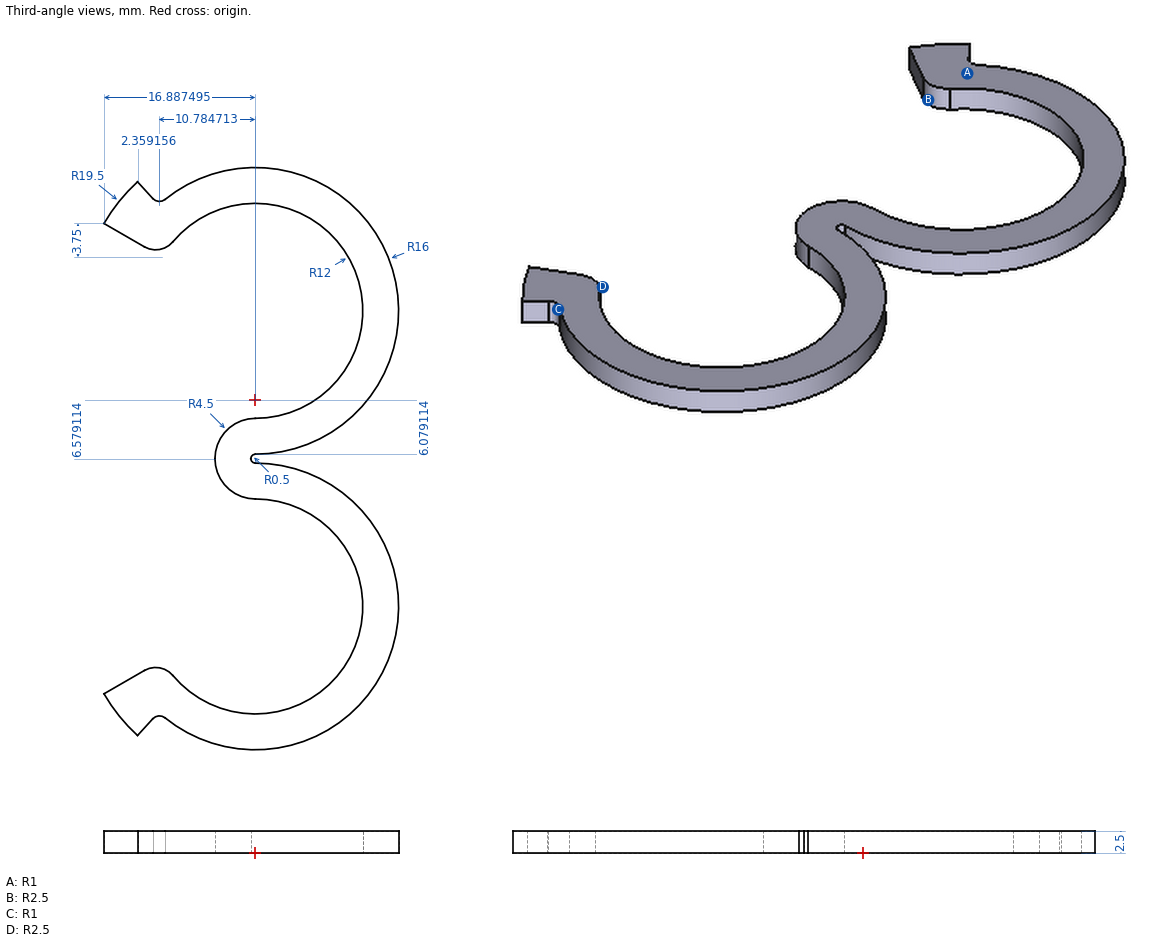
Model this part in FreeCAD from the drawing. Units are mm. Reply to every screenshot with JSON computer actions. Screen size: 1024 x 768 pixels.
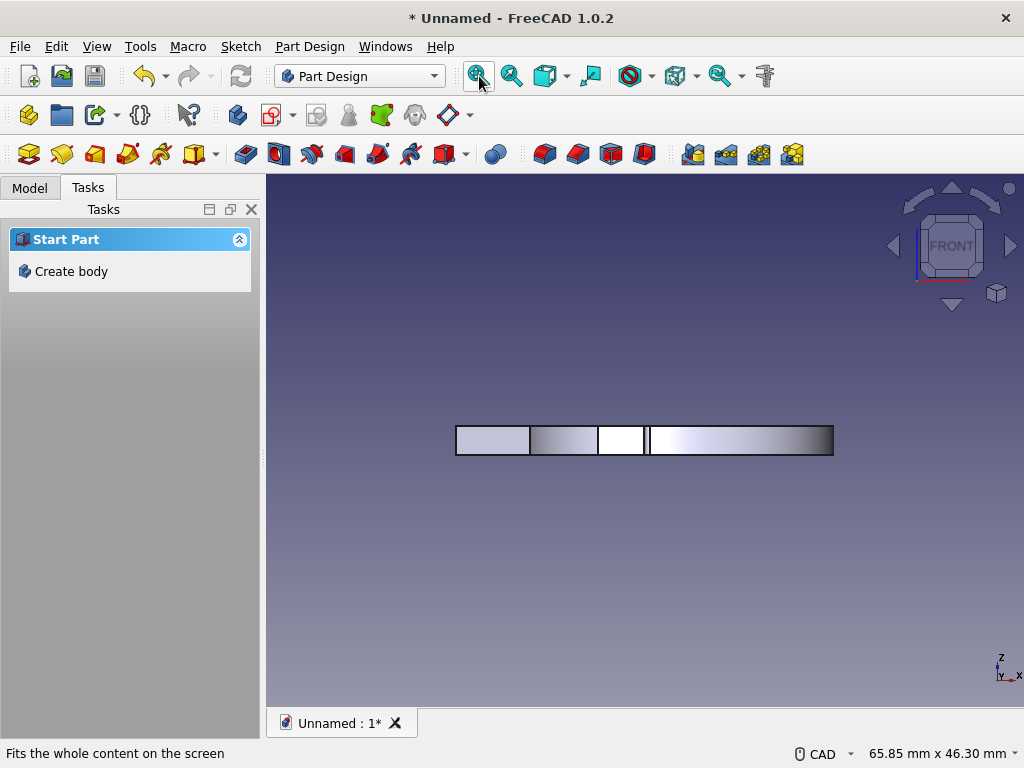
{"action": "key", "text": "3"}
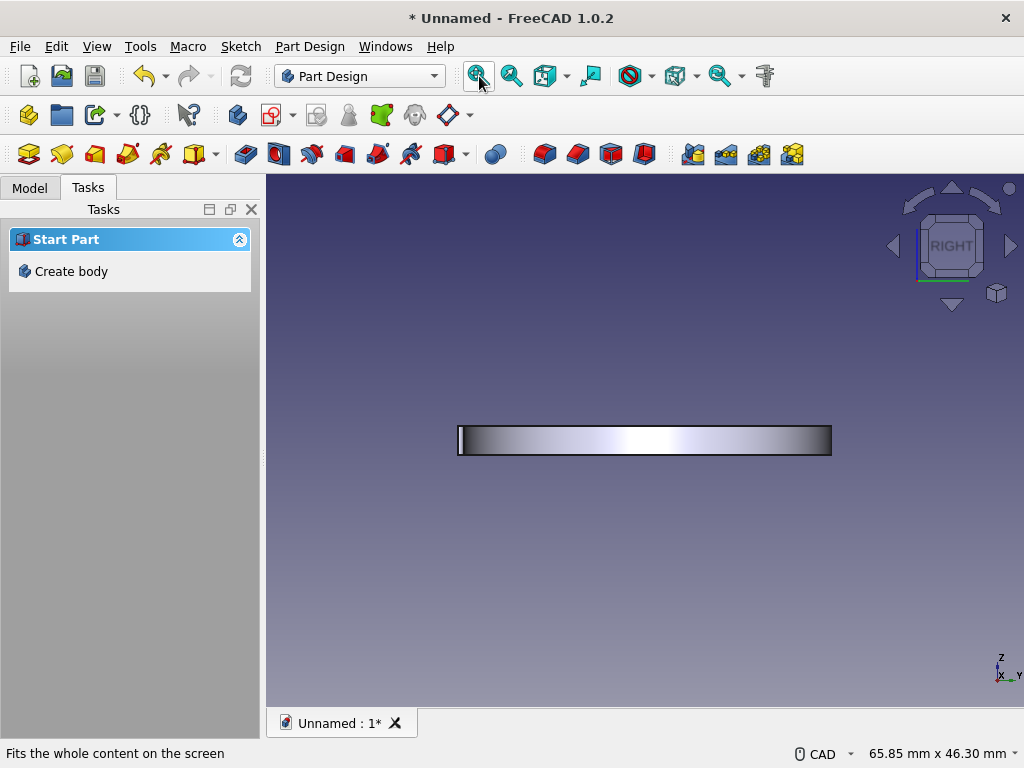
{"action": "key", "text": "5"}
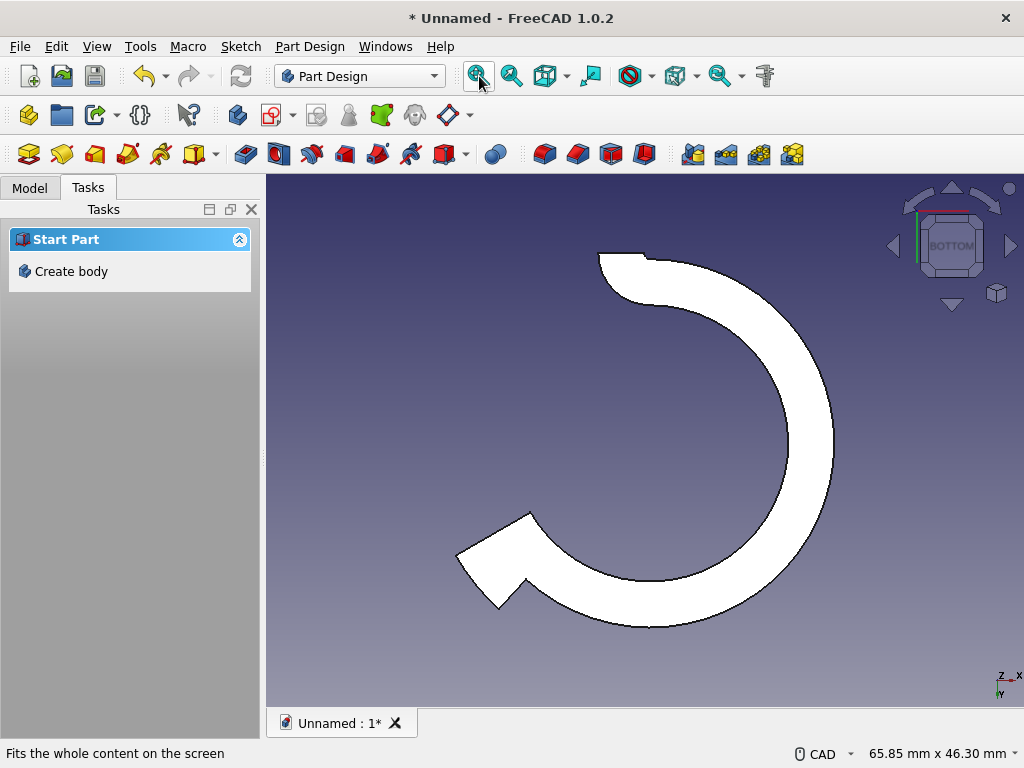
{"action": "key", "text": "4"}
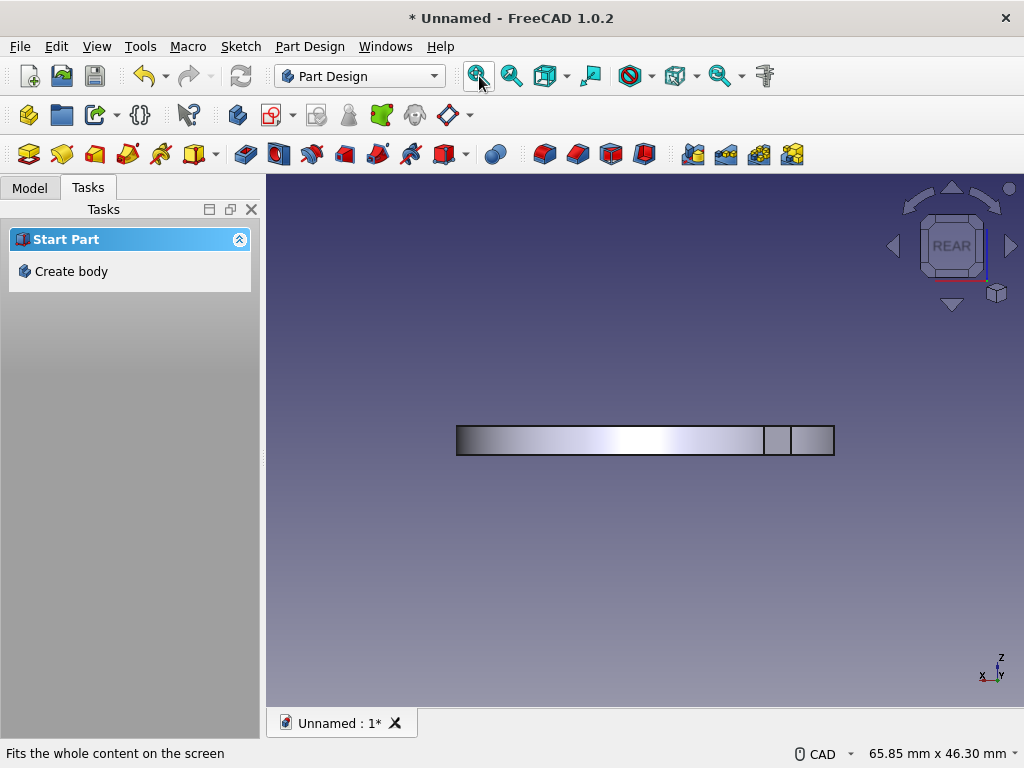
{"action": "key", "text": "6"}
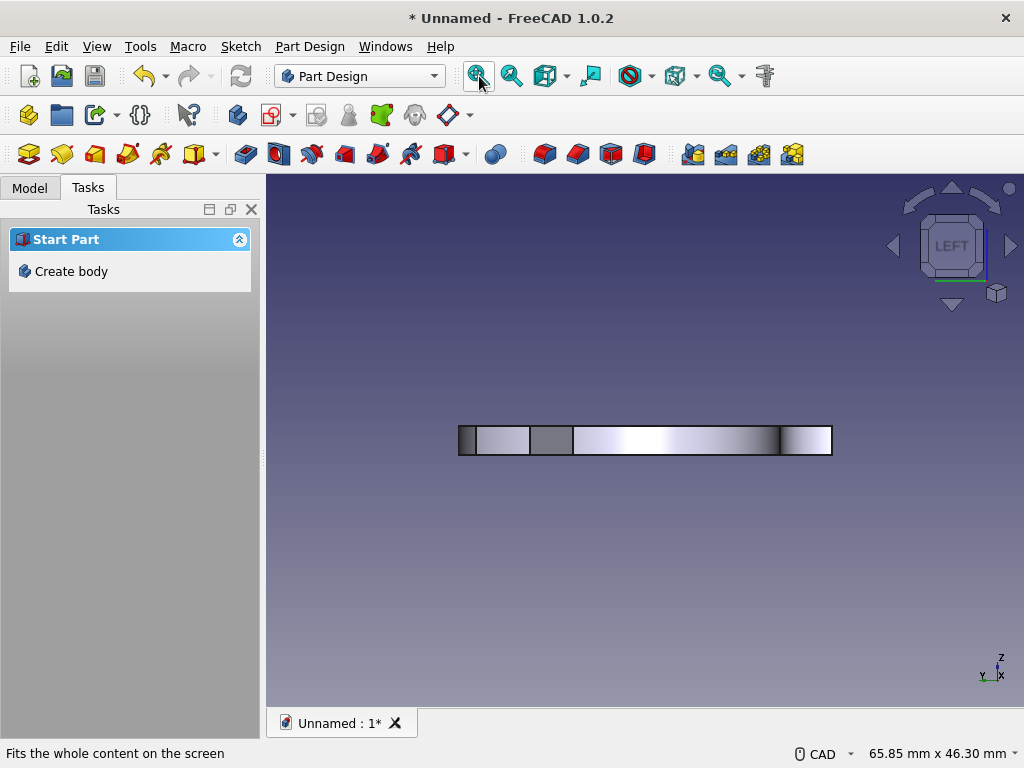
{"action": "key", "text": "v 3"}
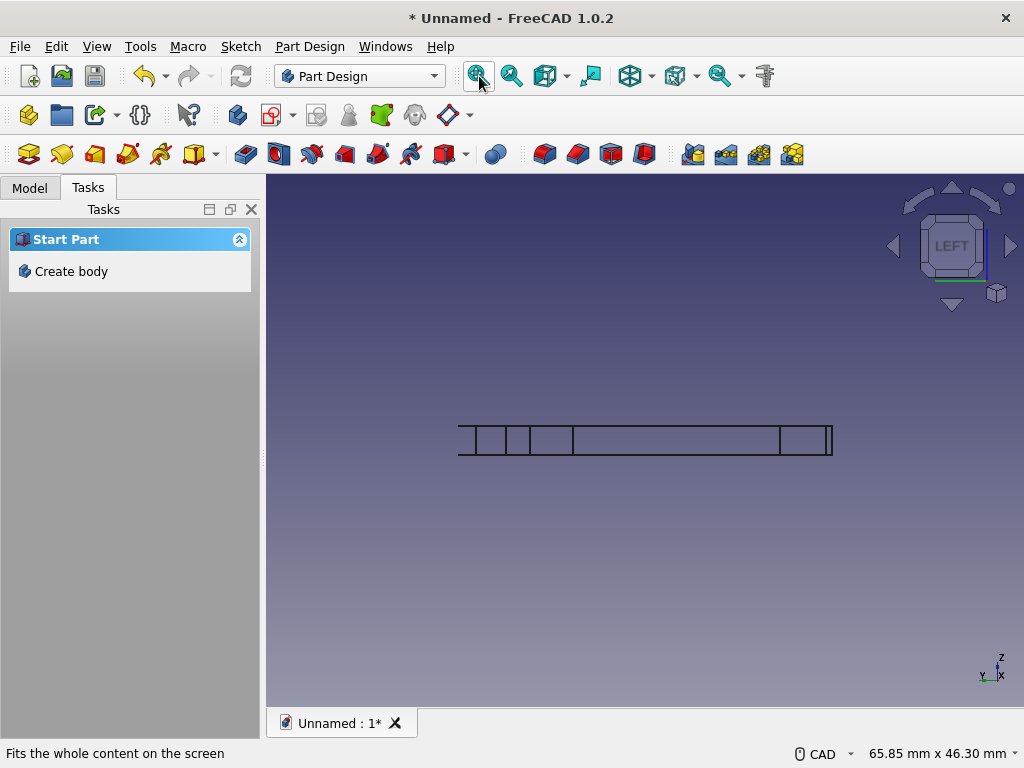
{"action": "key", "text": "0"}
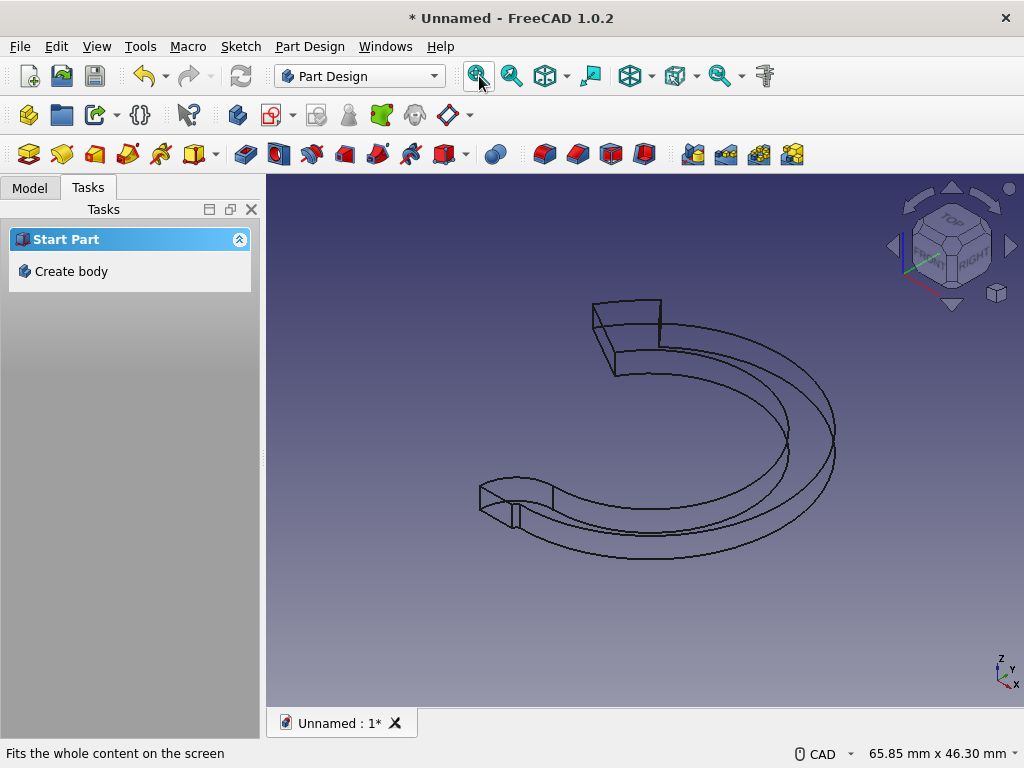
{"action": "left_click", "coordinate": [659, 334]}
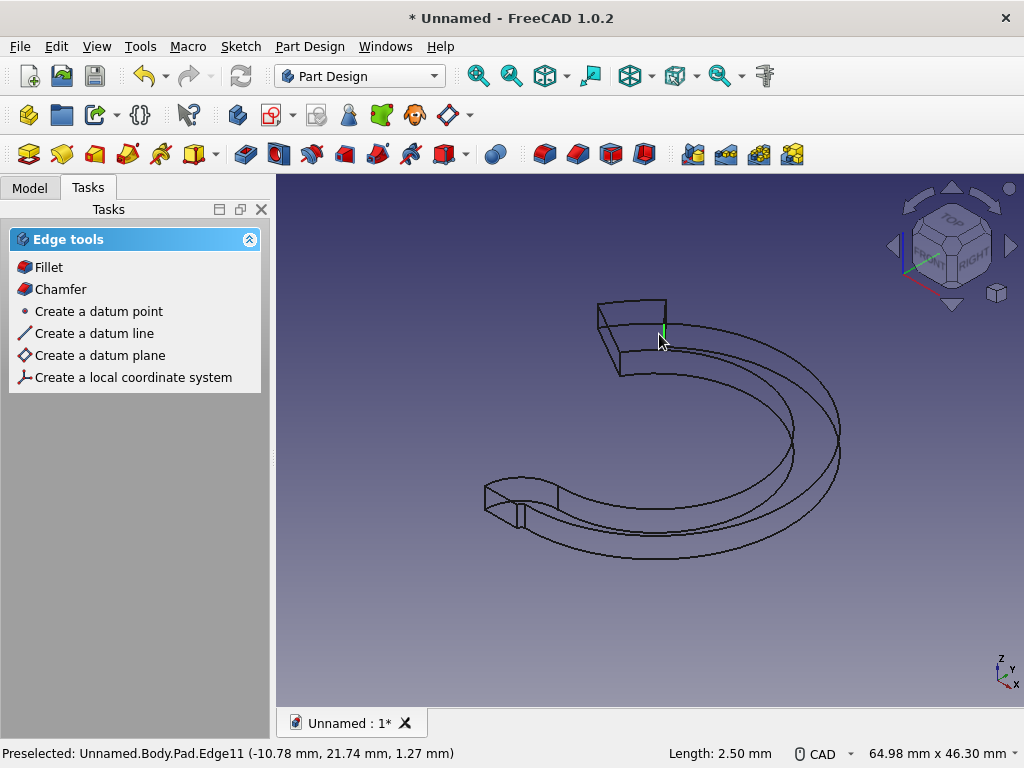
{"action": "key", "text": "v 1"}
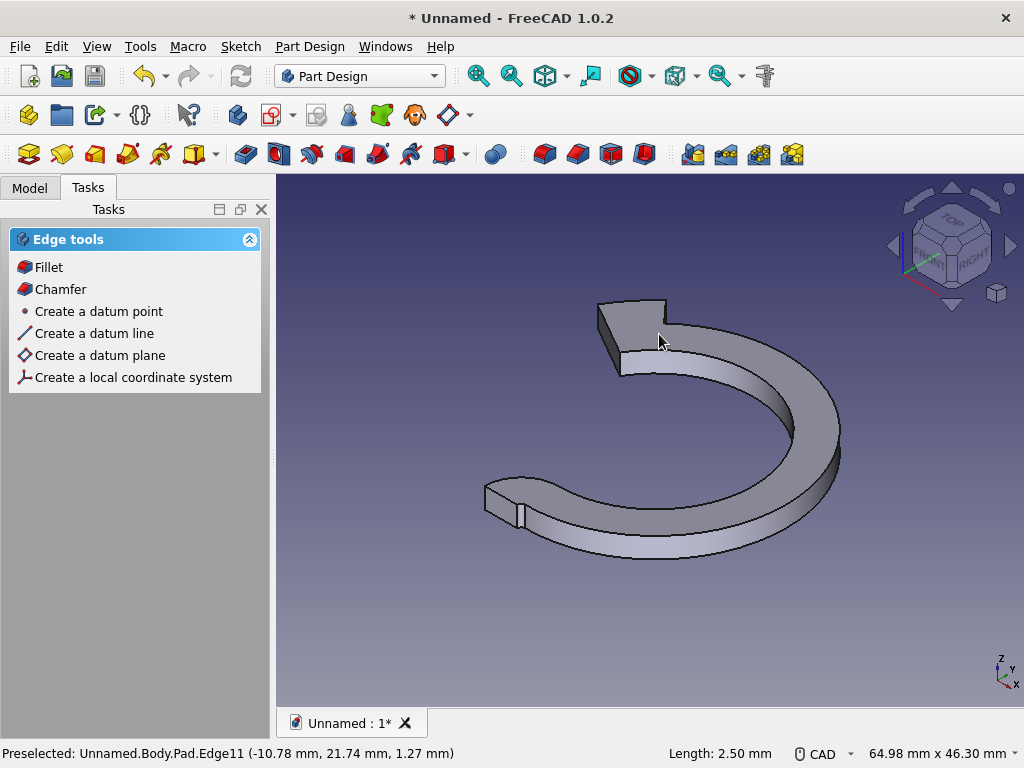
{"action": "left_click", "coordinate": [545, 154]}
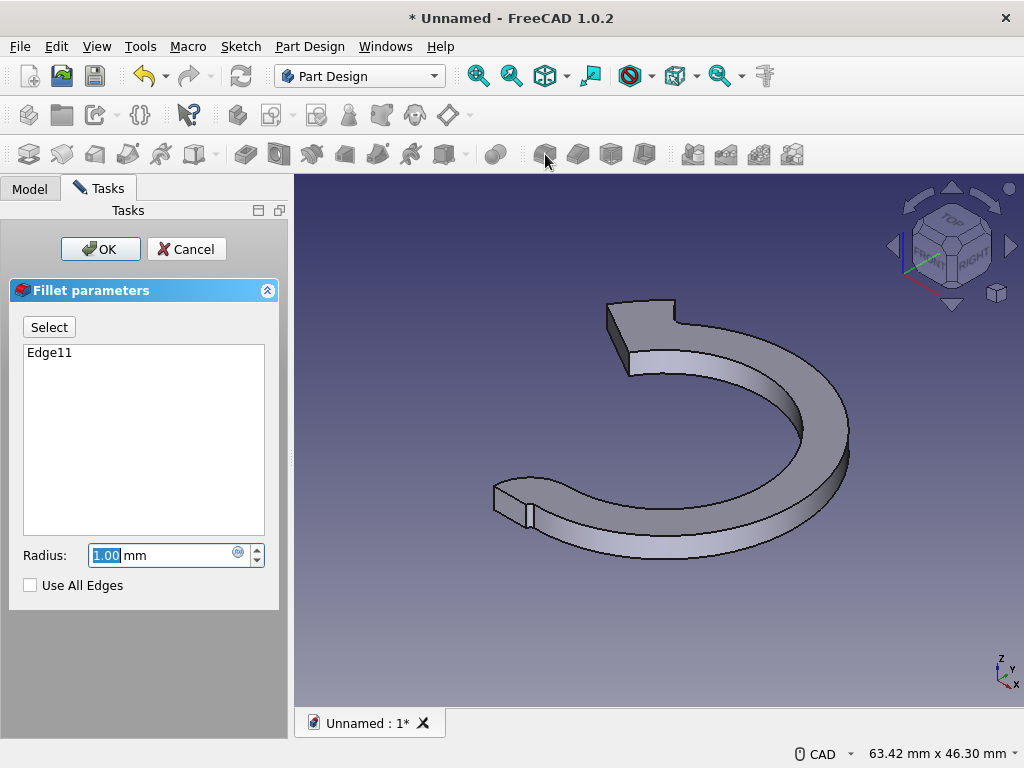
{"action": "type", "text": "1"}
{"action": "key", "text": "Tab"}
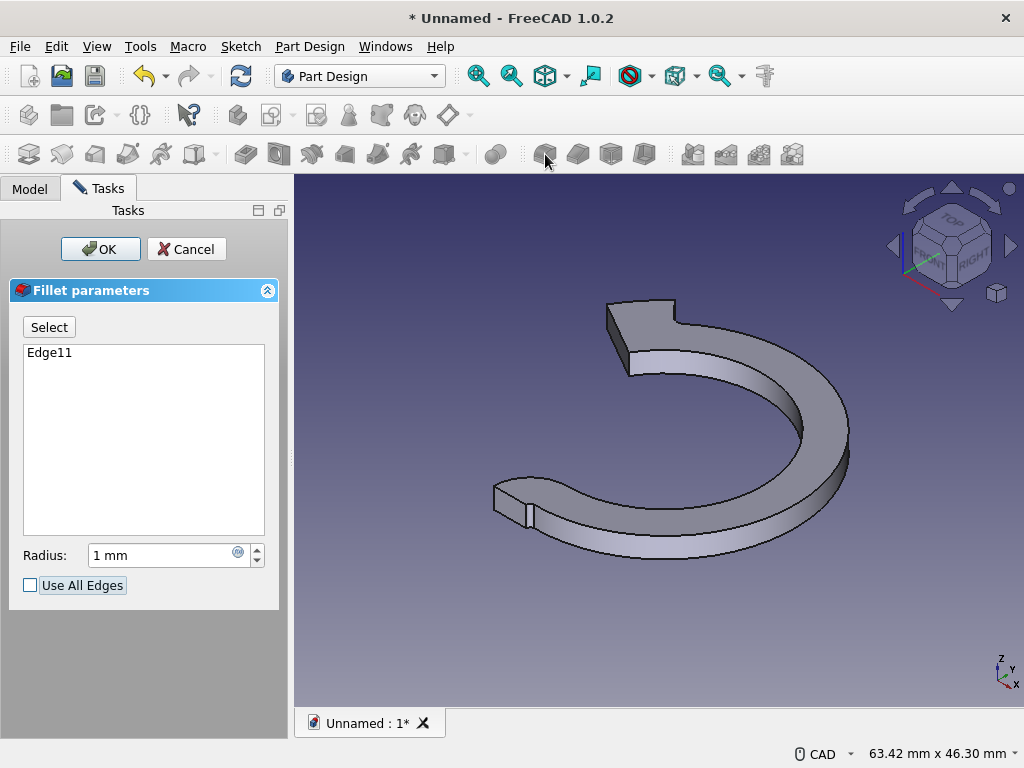
{"action": "left_click", "coordinate": [101, 249]}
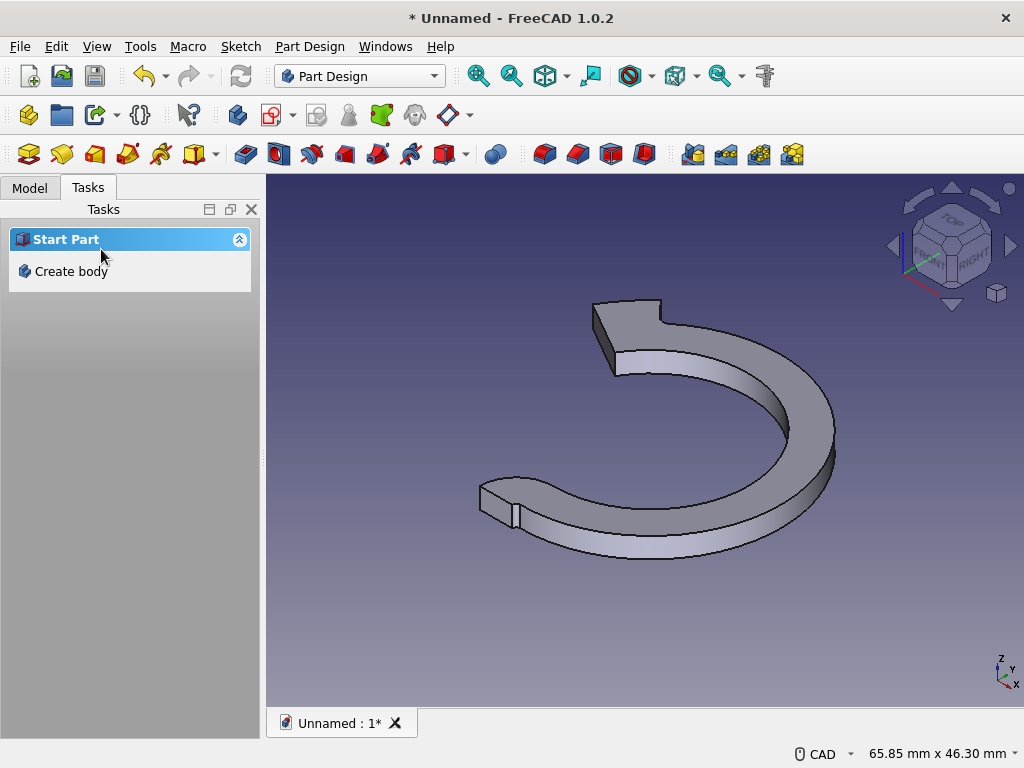
{"action": "left_click", "coordinate": [615, 363]}